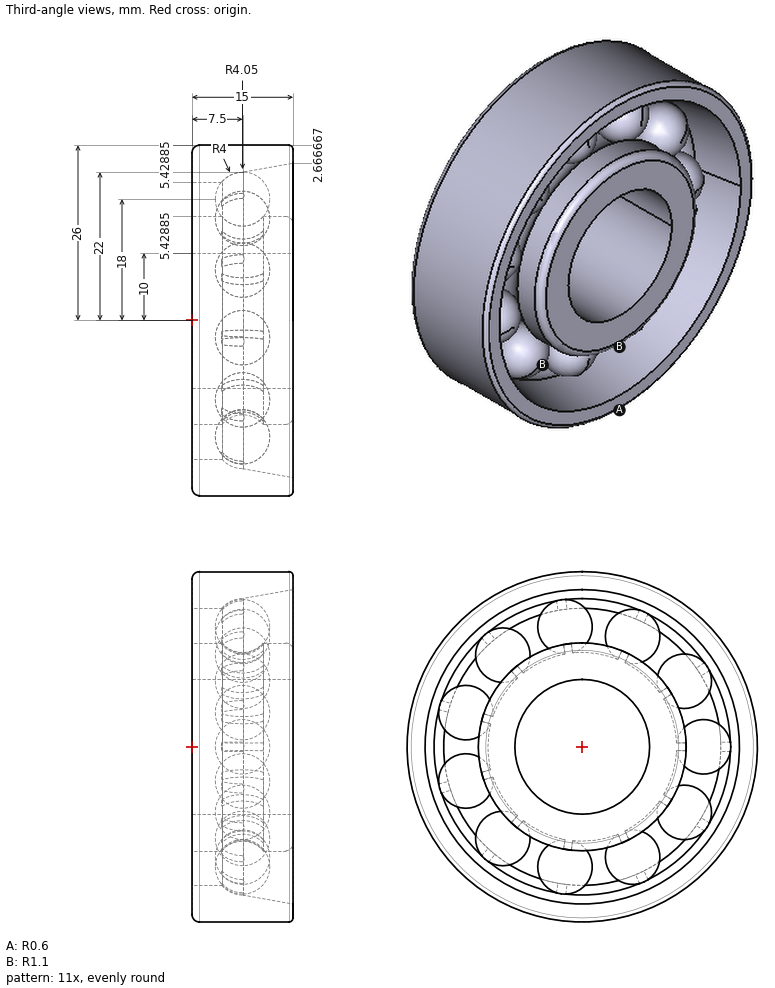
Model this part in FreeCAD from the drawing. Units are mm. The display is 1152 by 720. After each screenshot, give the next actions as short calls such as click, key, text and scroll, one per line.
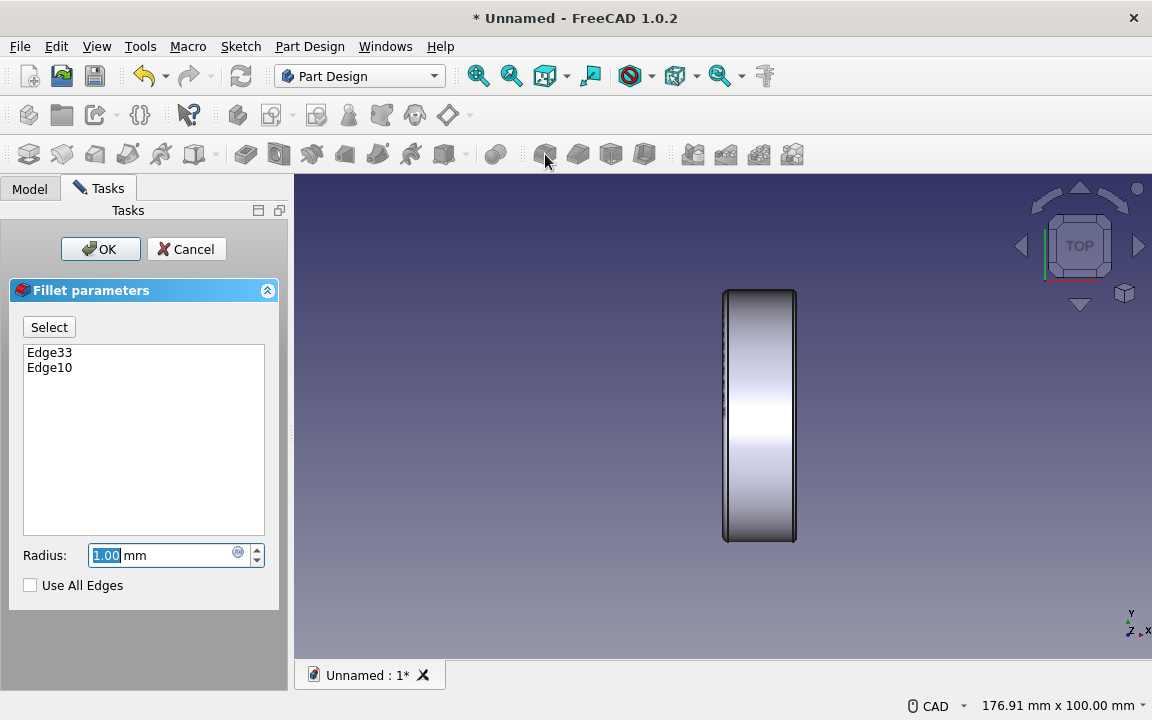
text(1.1)
key(Tab)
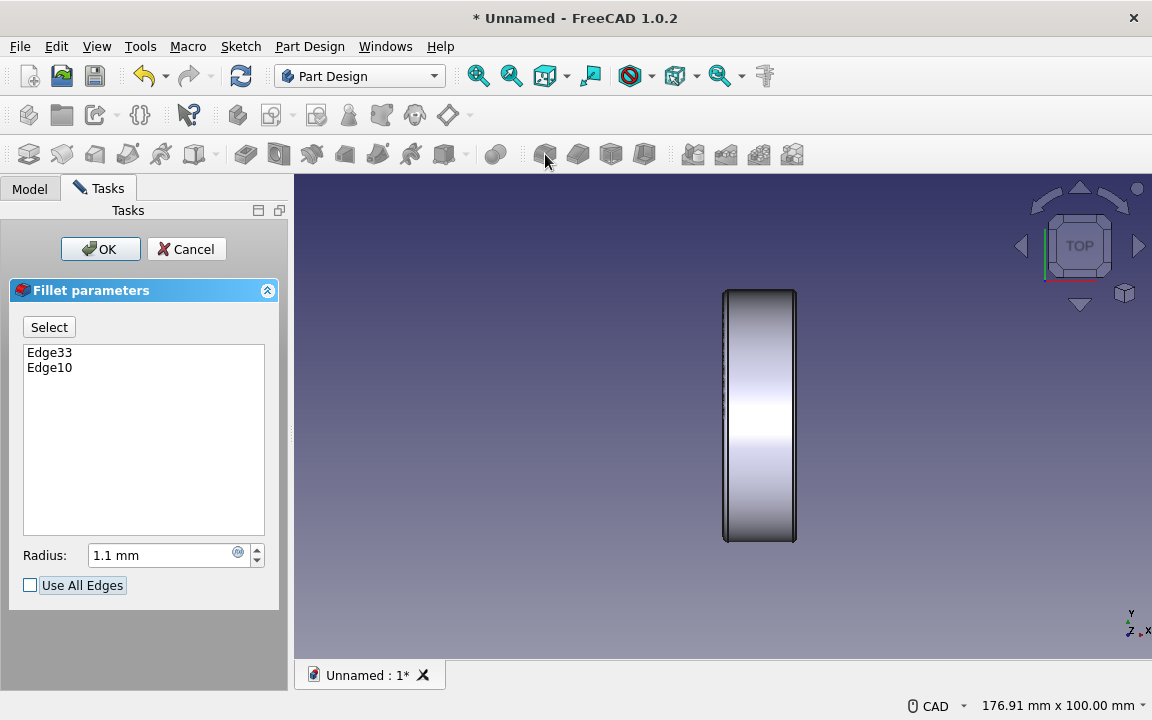
click(101, 249)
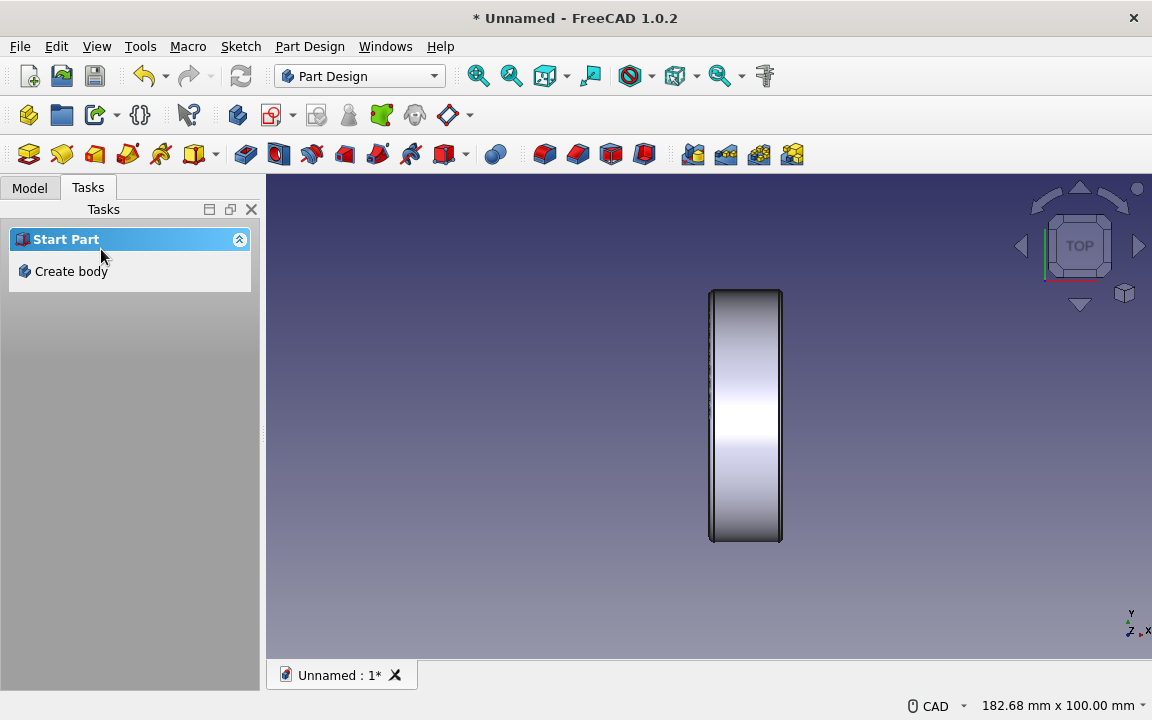
click(30, 188)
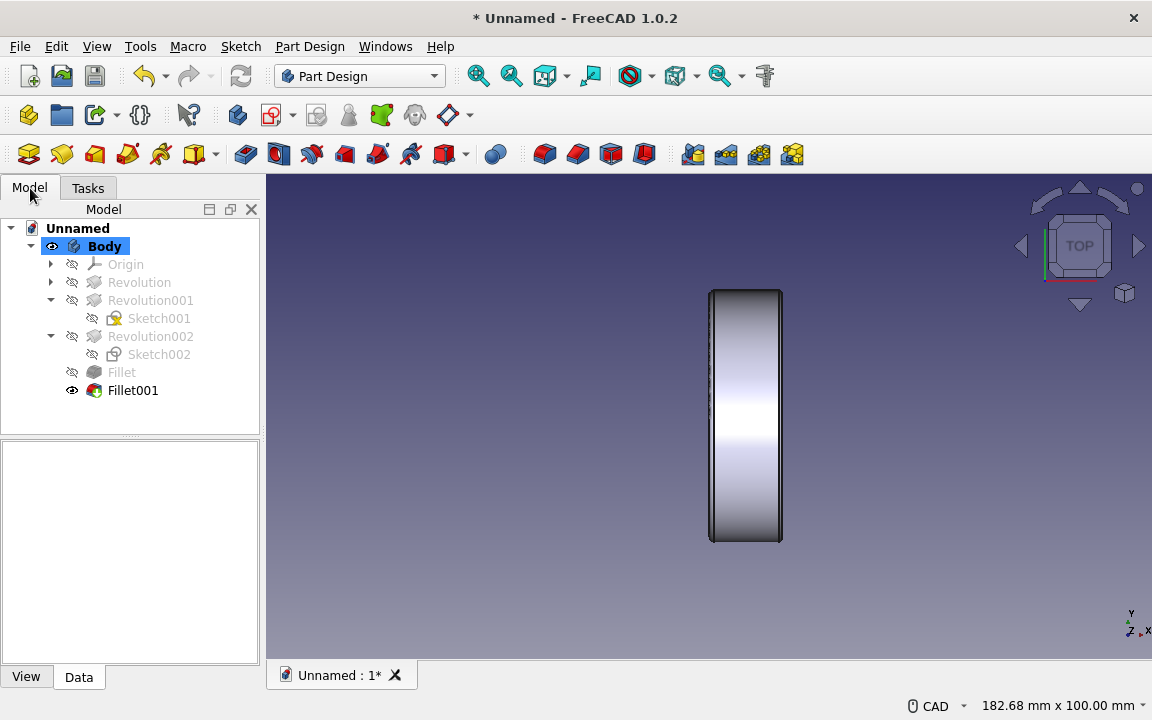
click(117, 300)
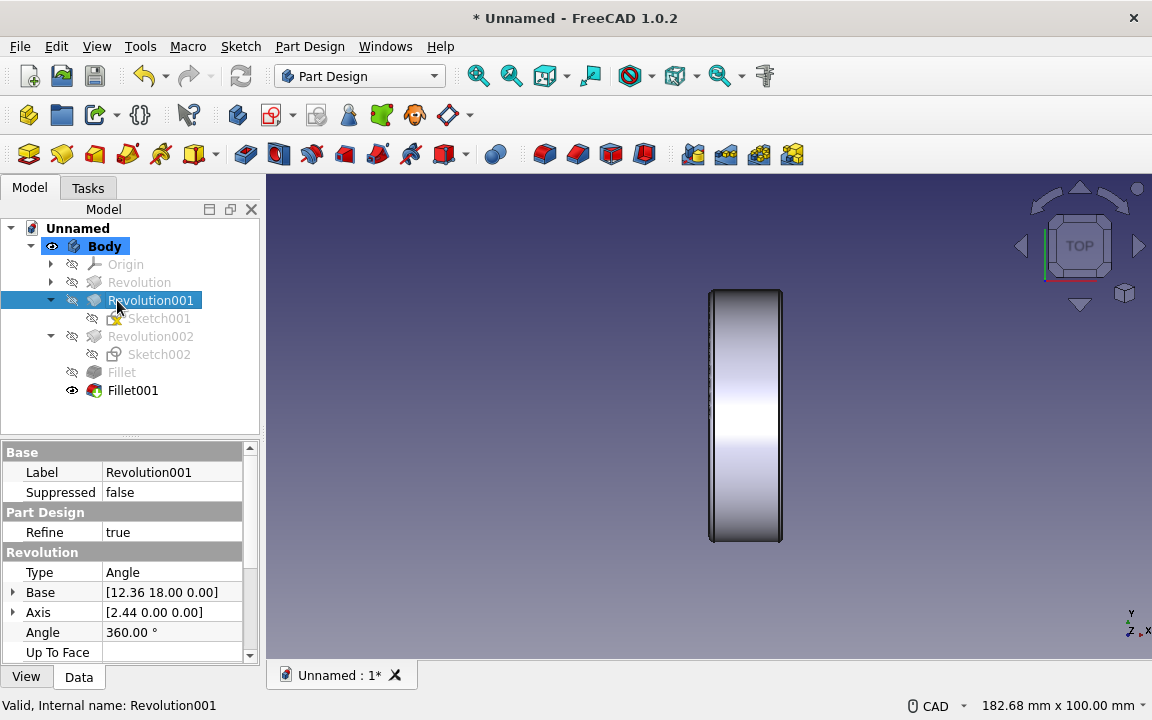
click(759, 154)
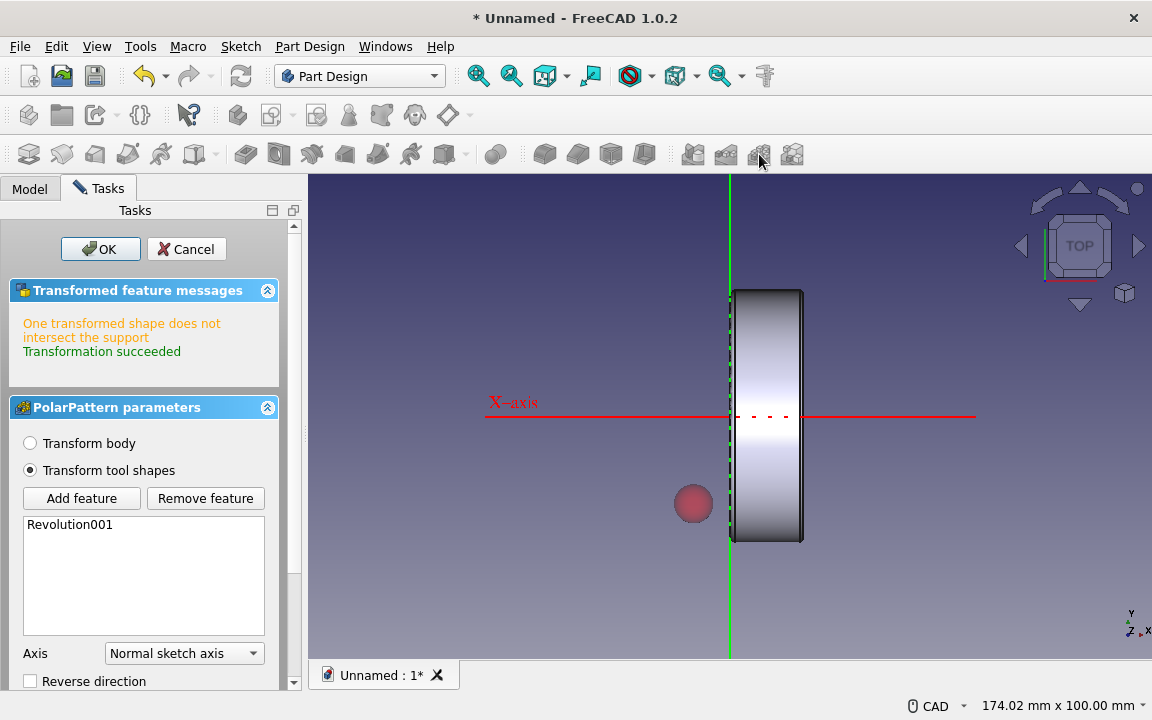
click(185, 654)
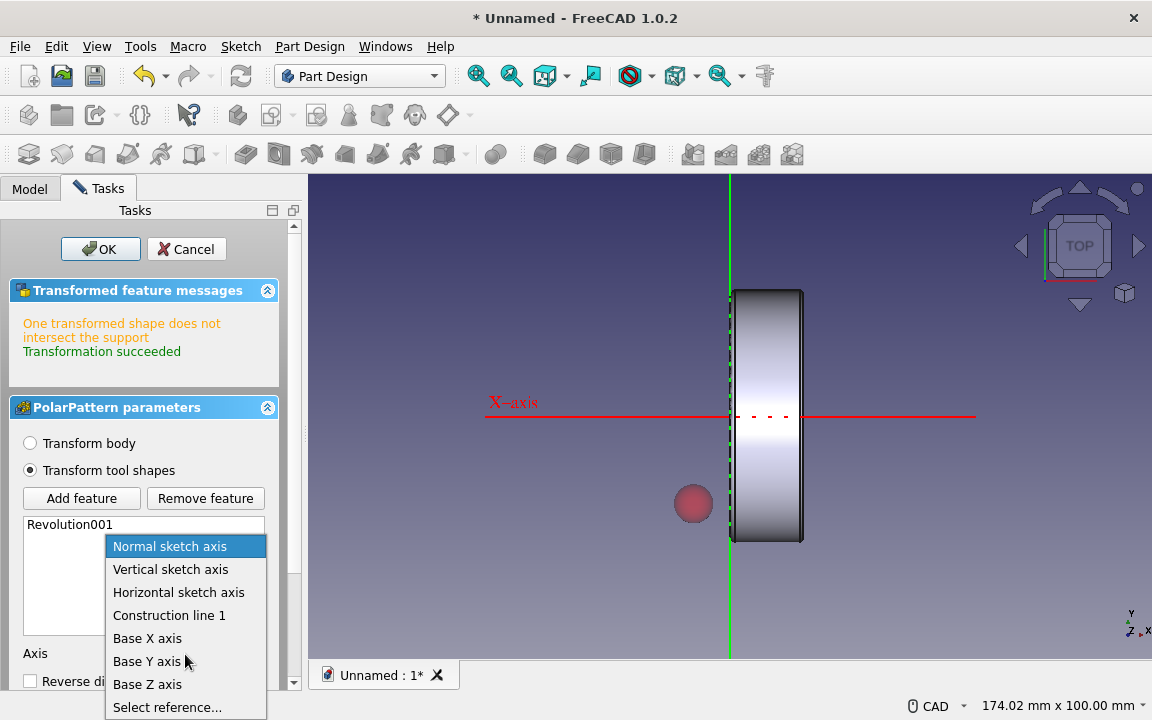
click(184, 638)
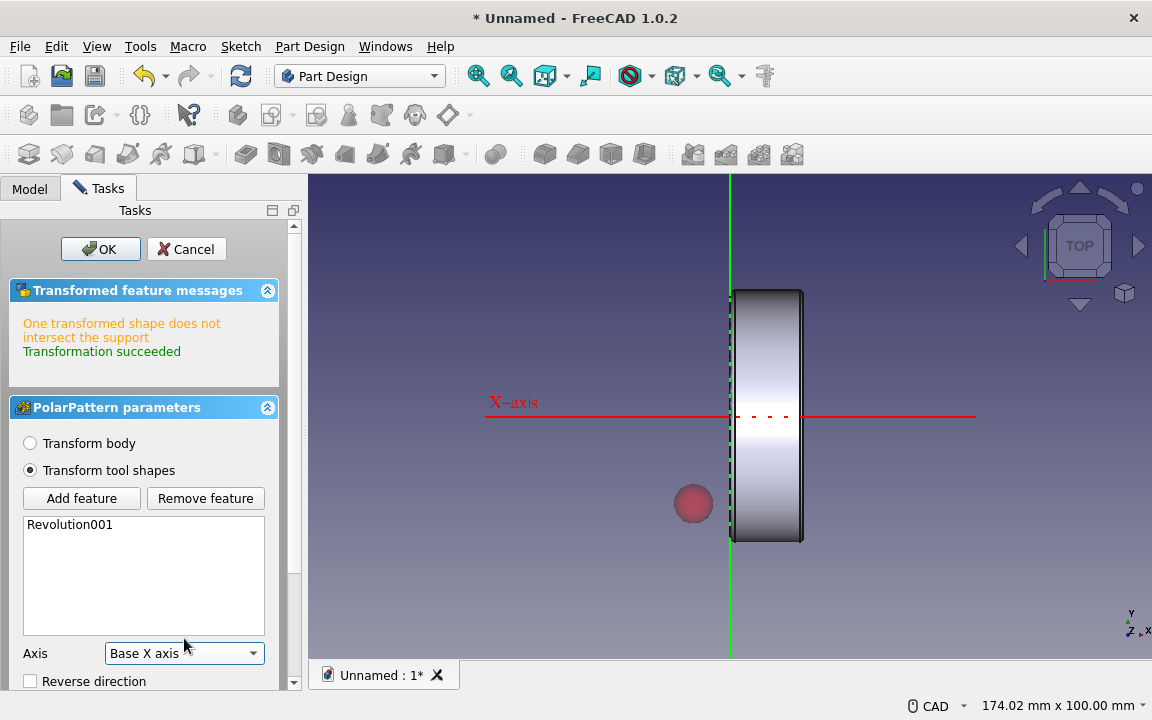
scroll(294, 455, down, 3)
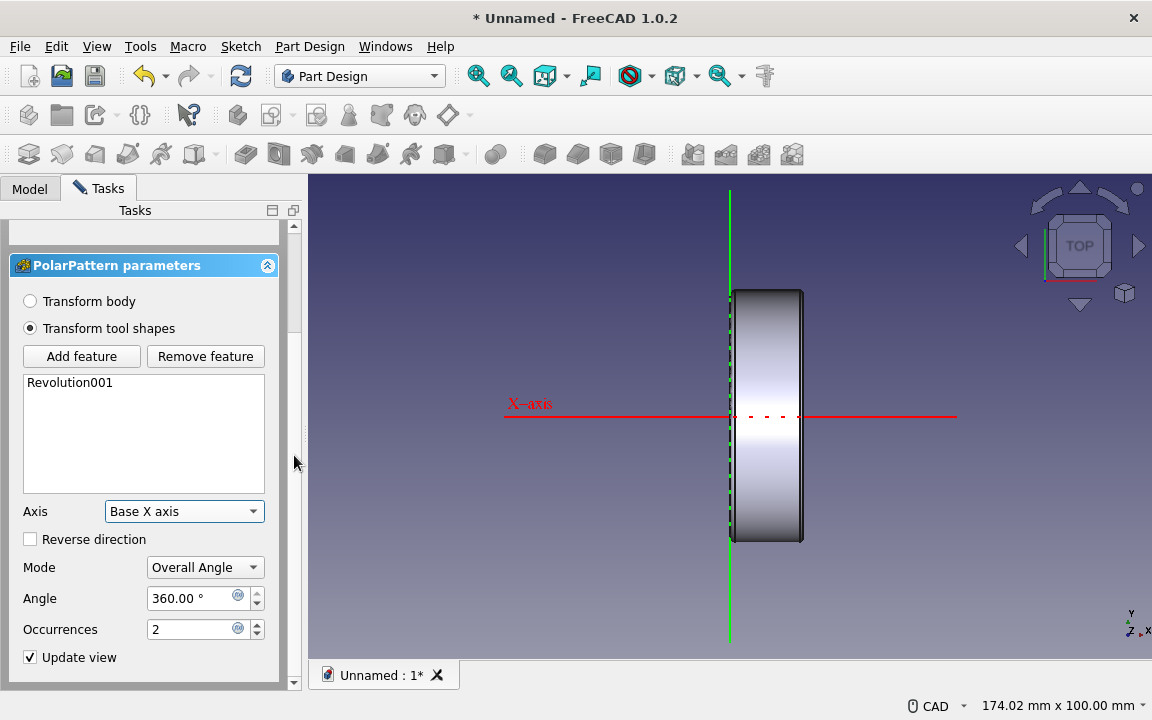
triple_click(199, 630)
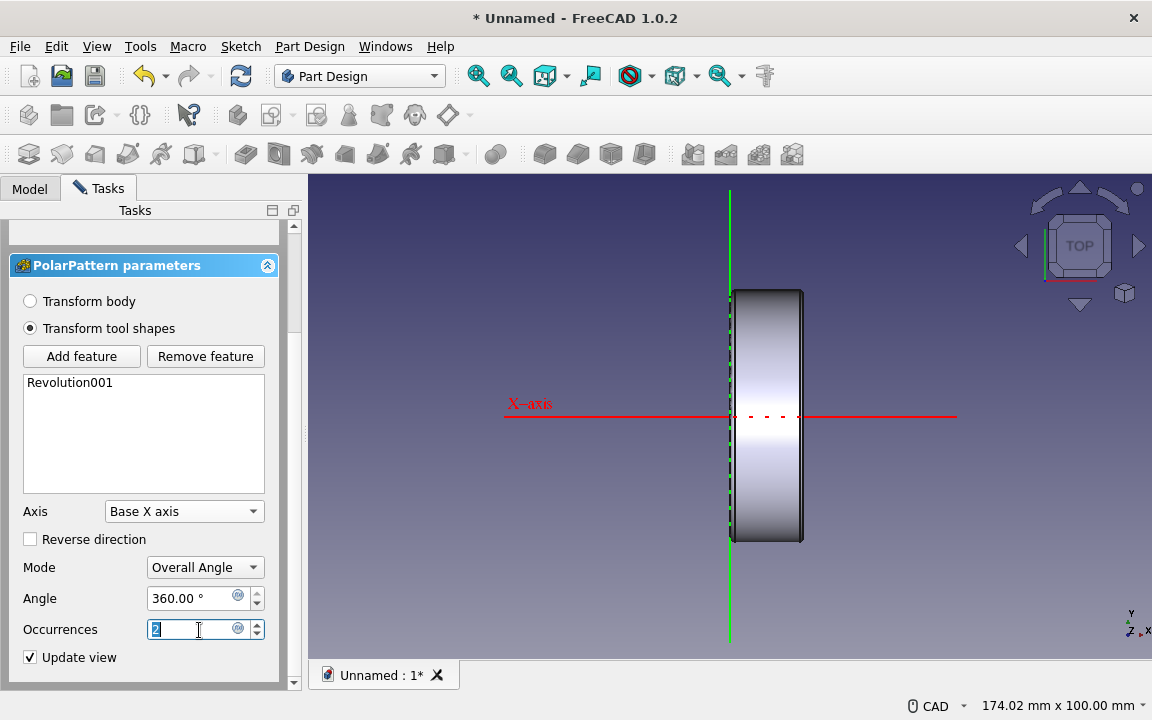
text(11)
key(Tab)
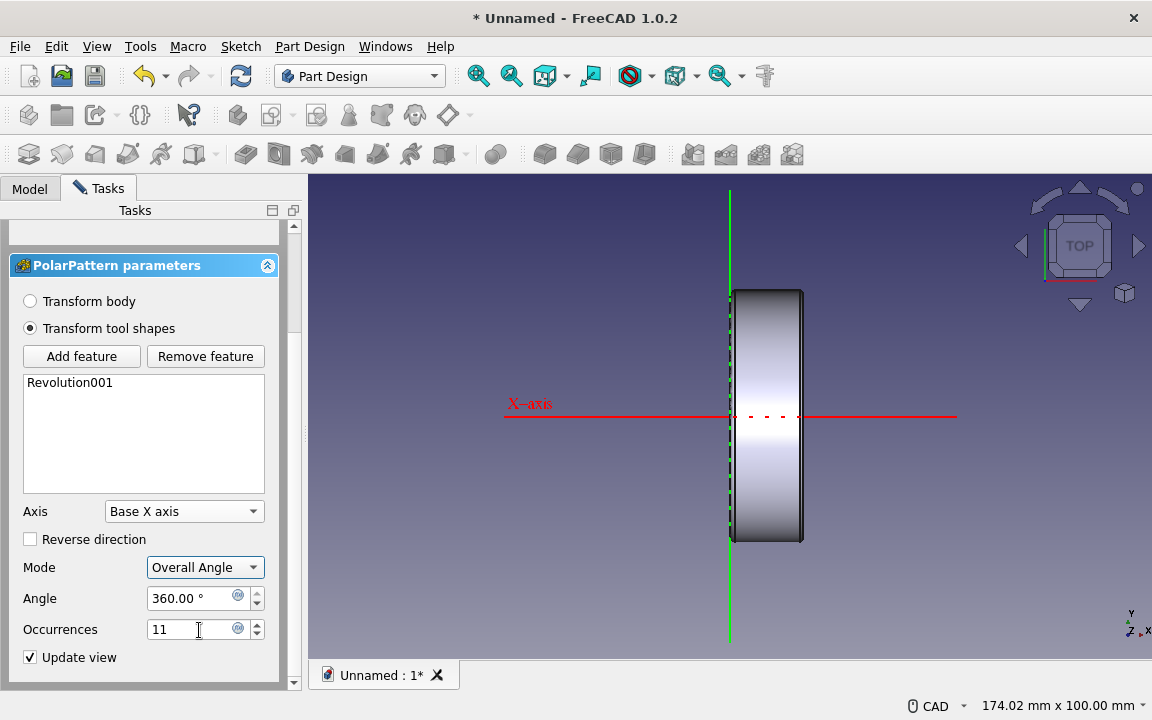
scroll(294, 455, up, 3)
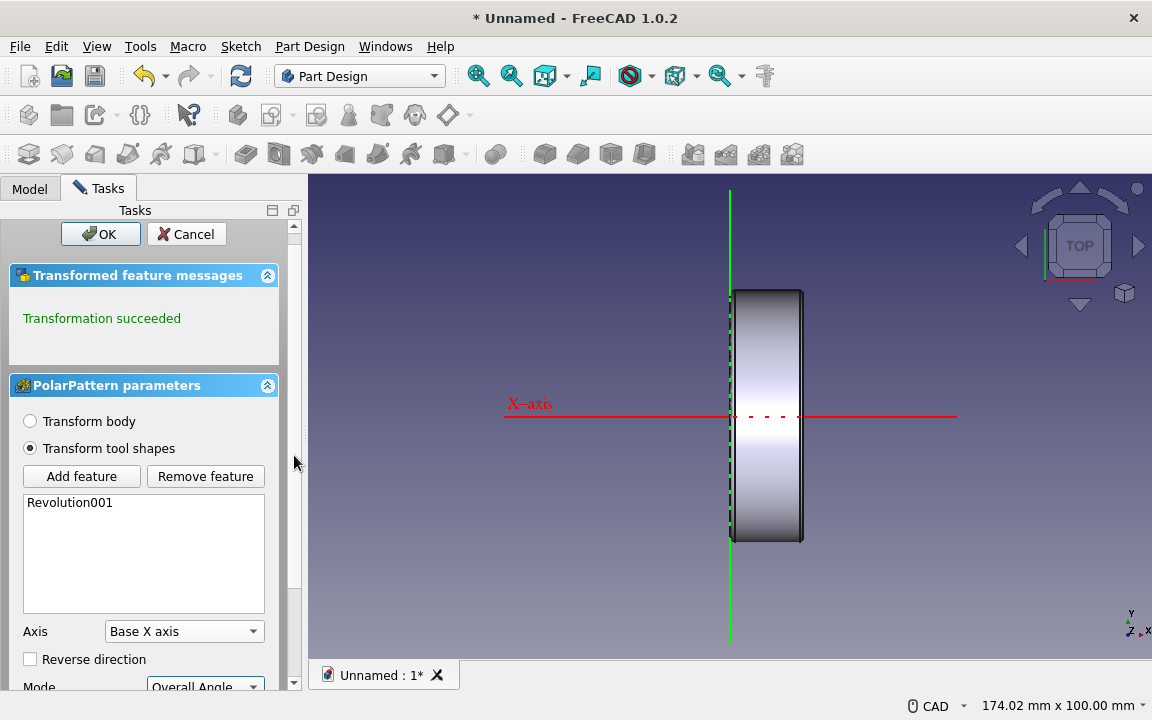
click(101, 249)